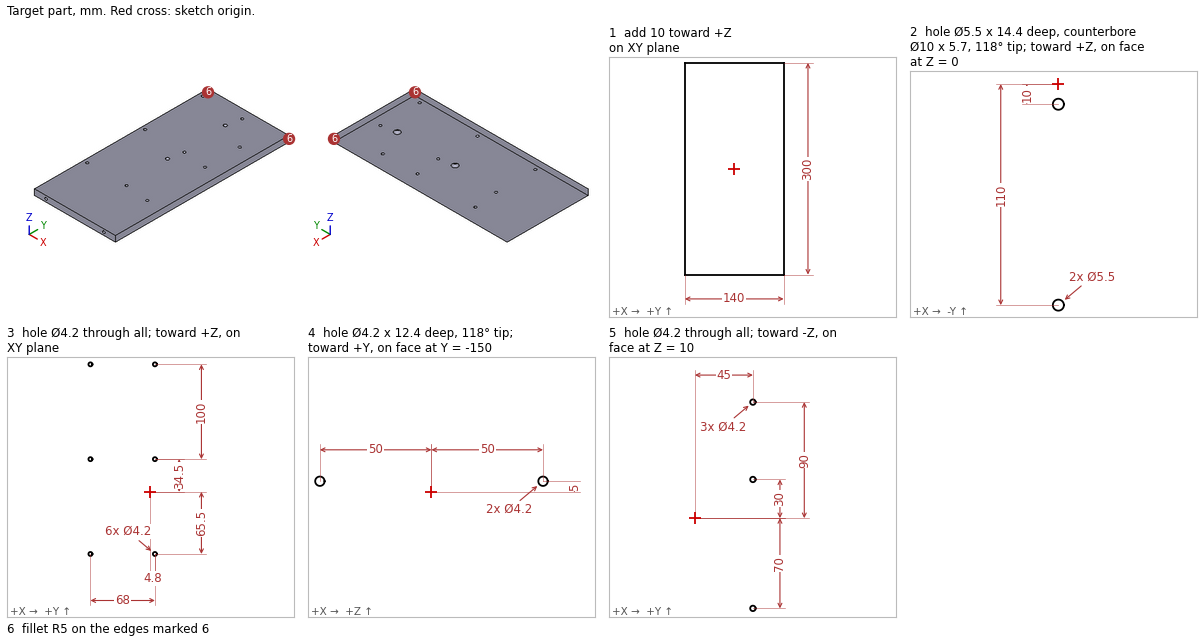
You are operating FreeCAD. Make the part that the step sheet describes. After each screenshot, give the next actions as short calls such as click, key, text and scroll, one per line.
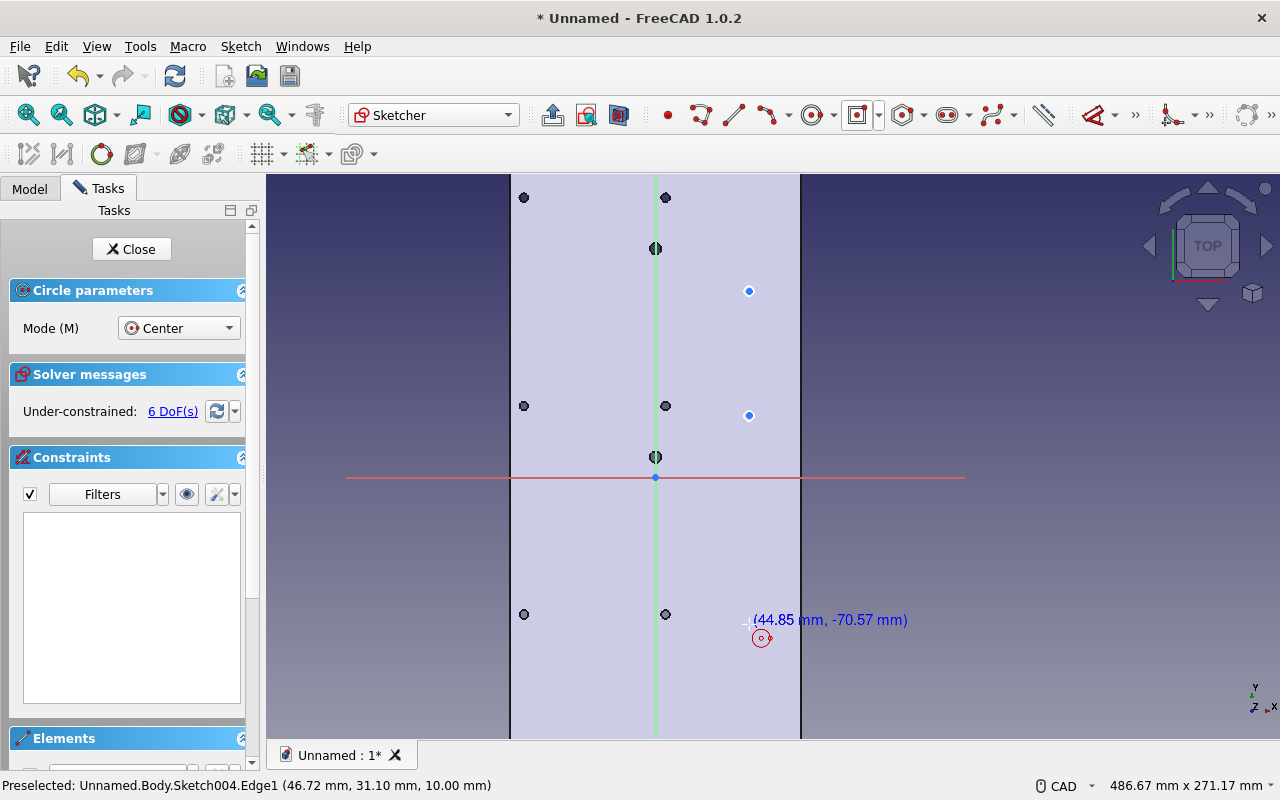
click(749, 624)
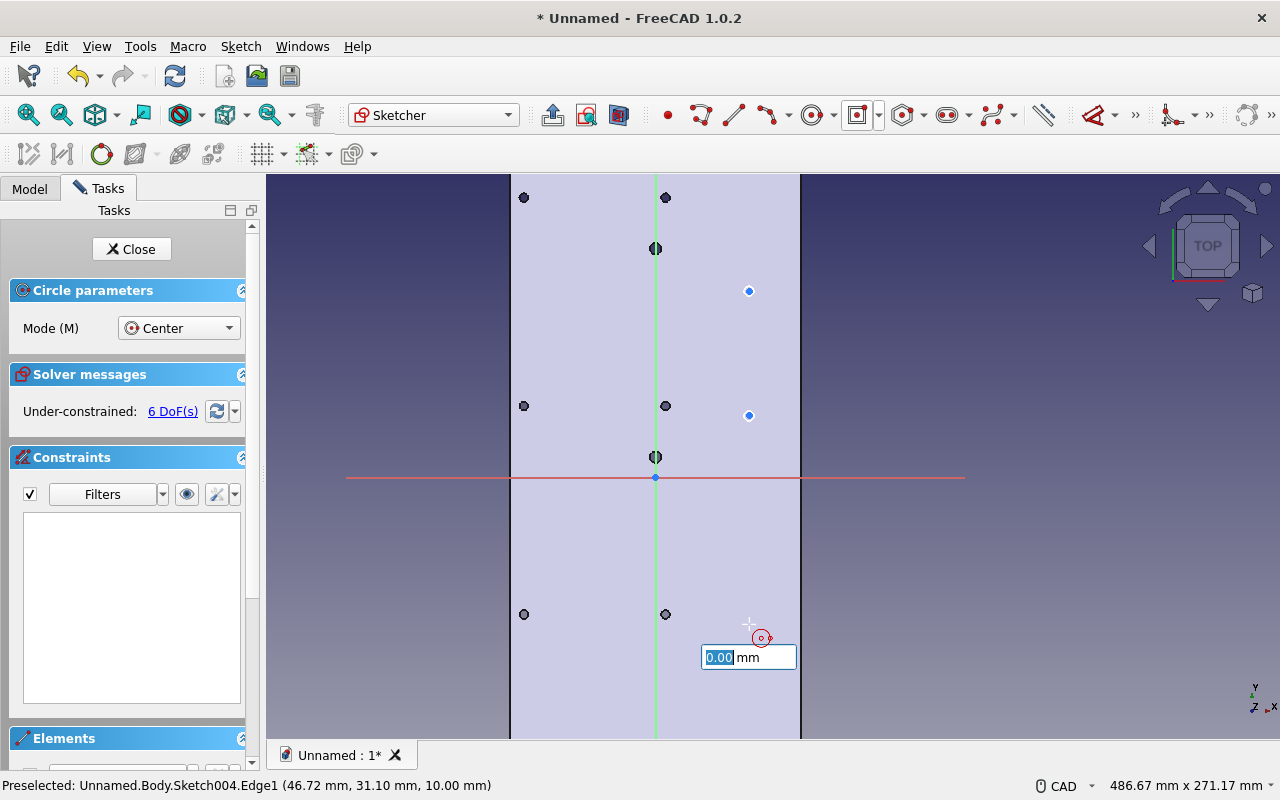
scroll(752, 621, up, 7)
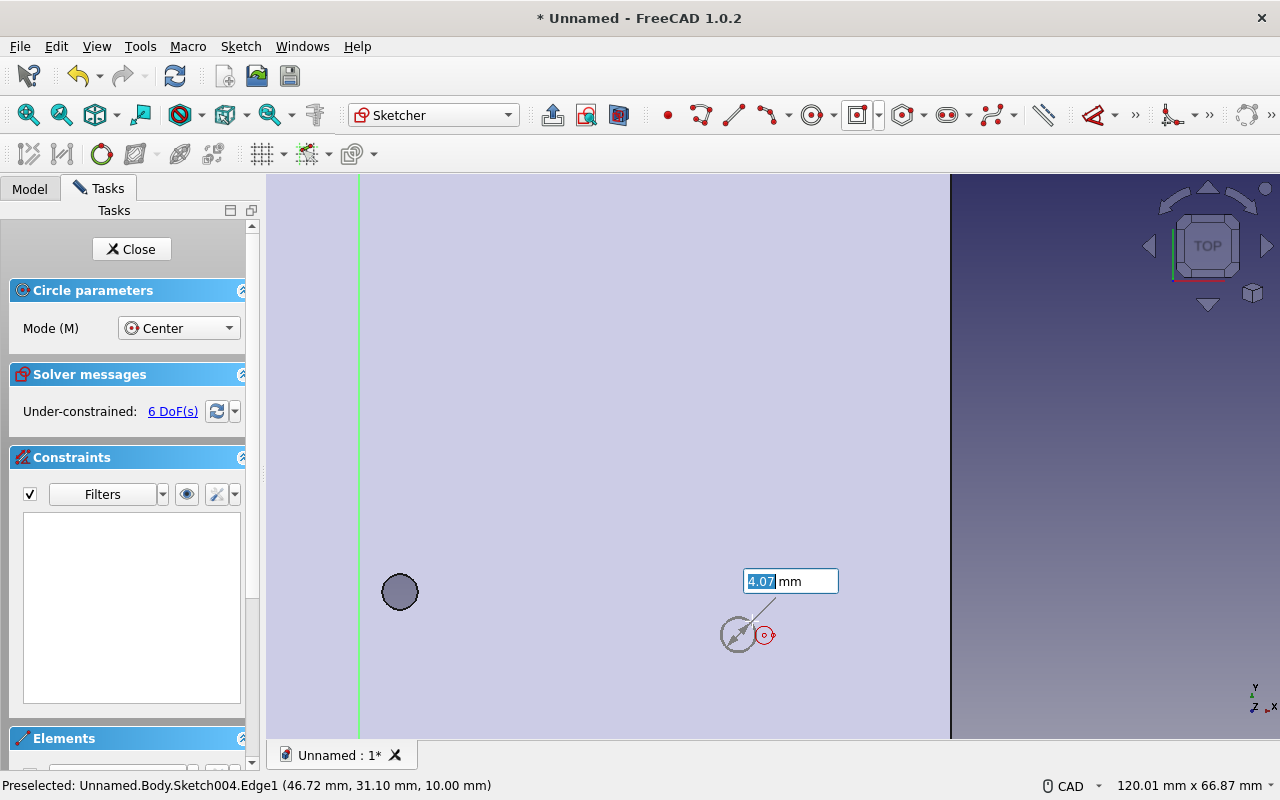
click(752, 617)
key(Escape)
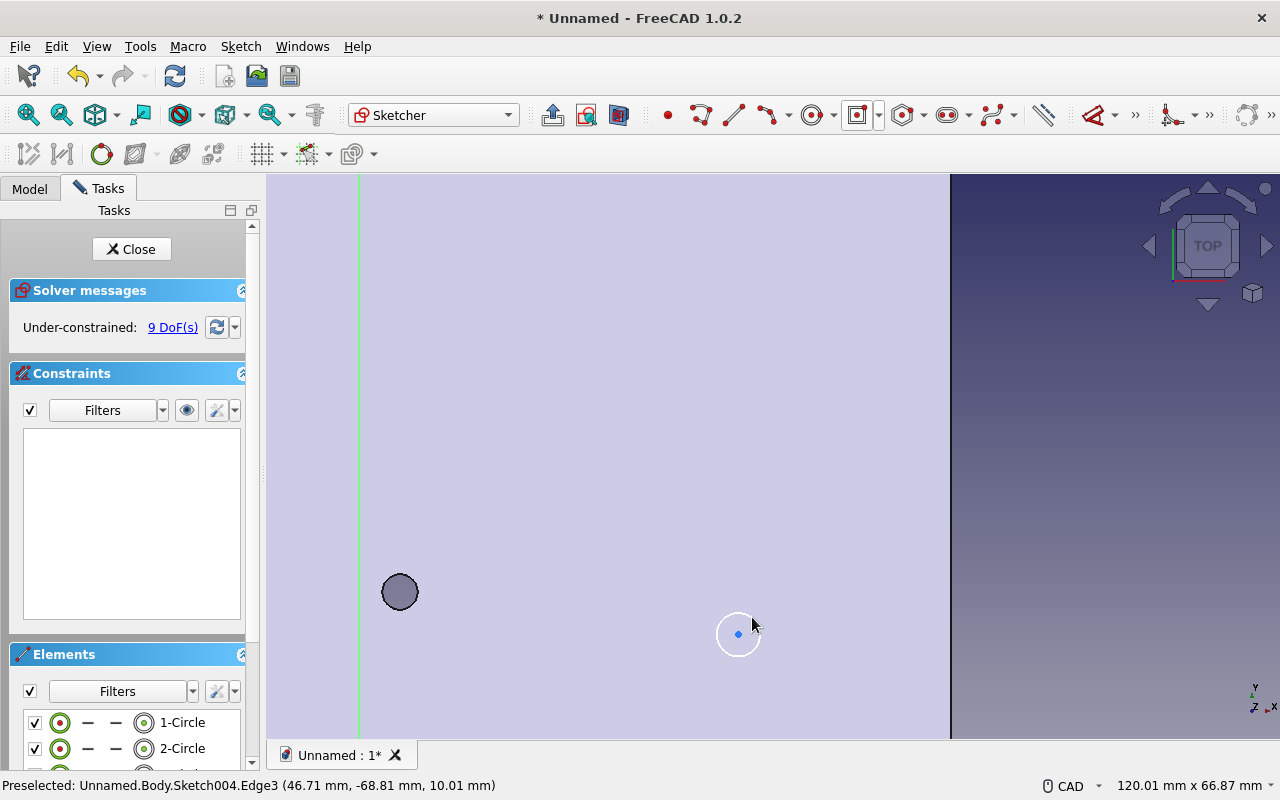
scroll(752, 621, down, 7)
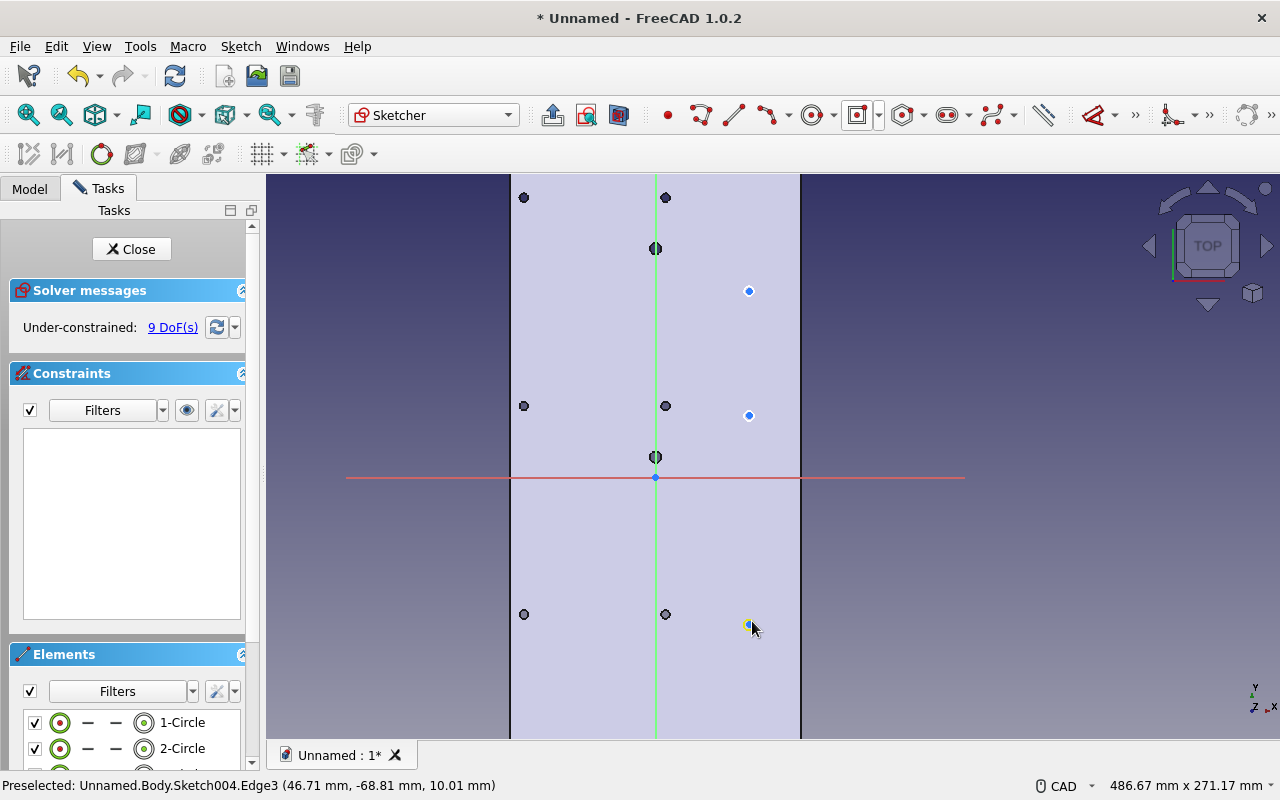
scroll(752, 288, up, 6)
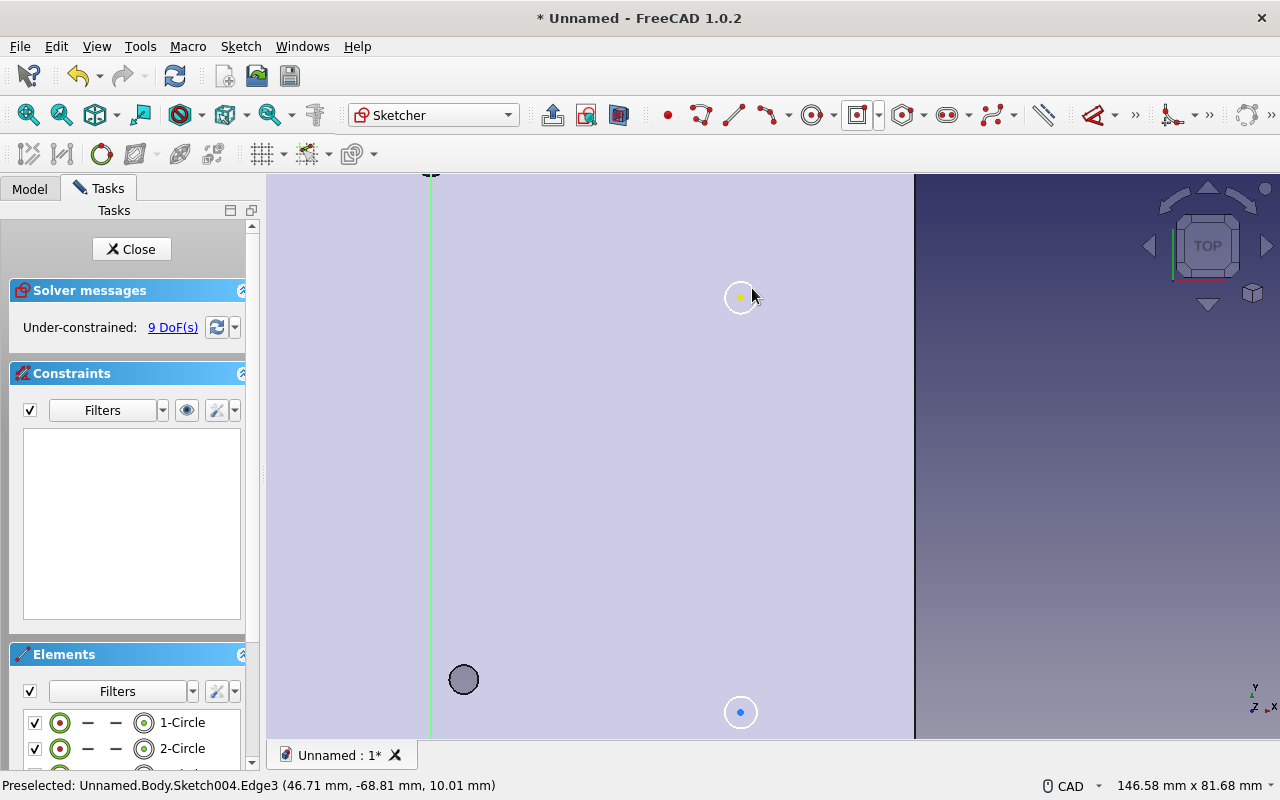
click(752, 287)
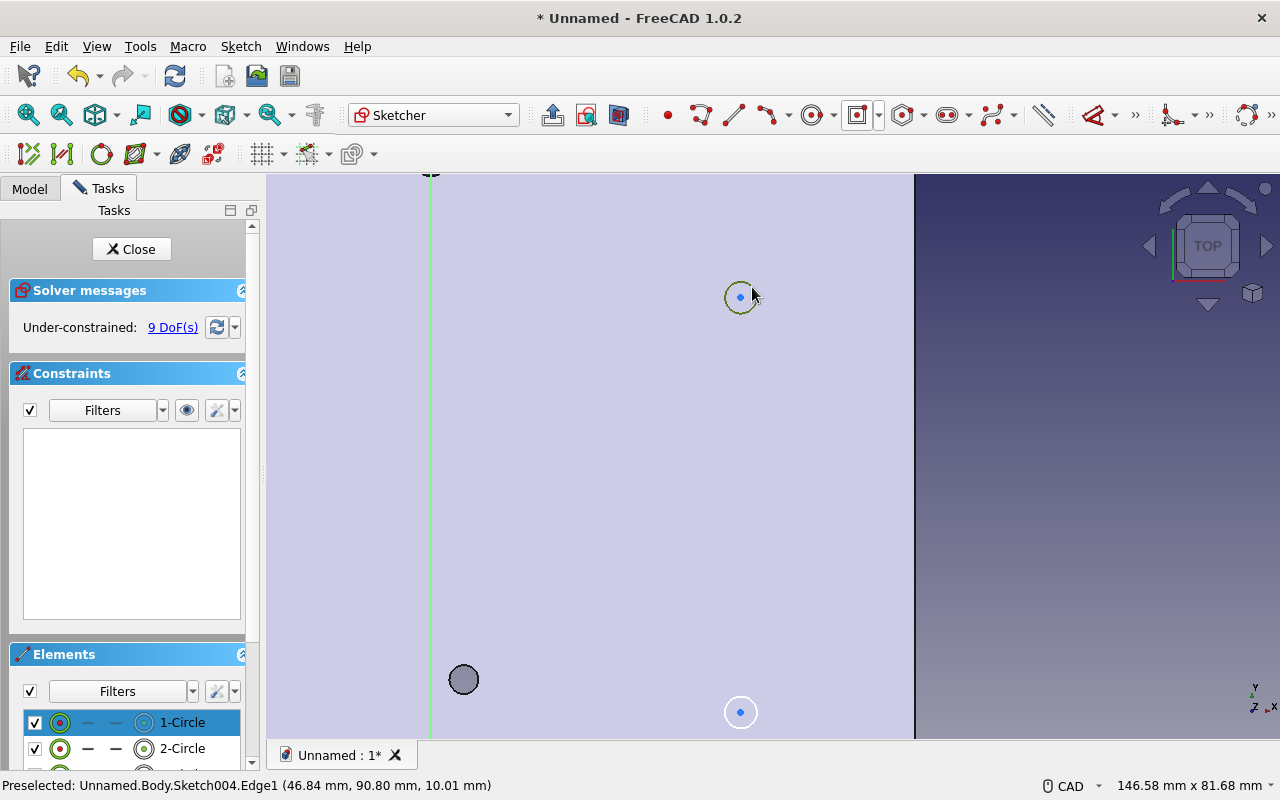
click(752, 701)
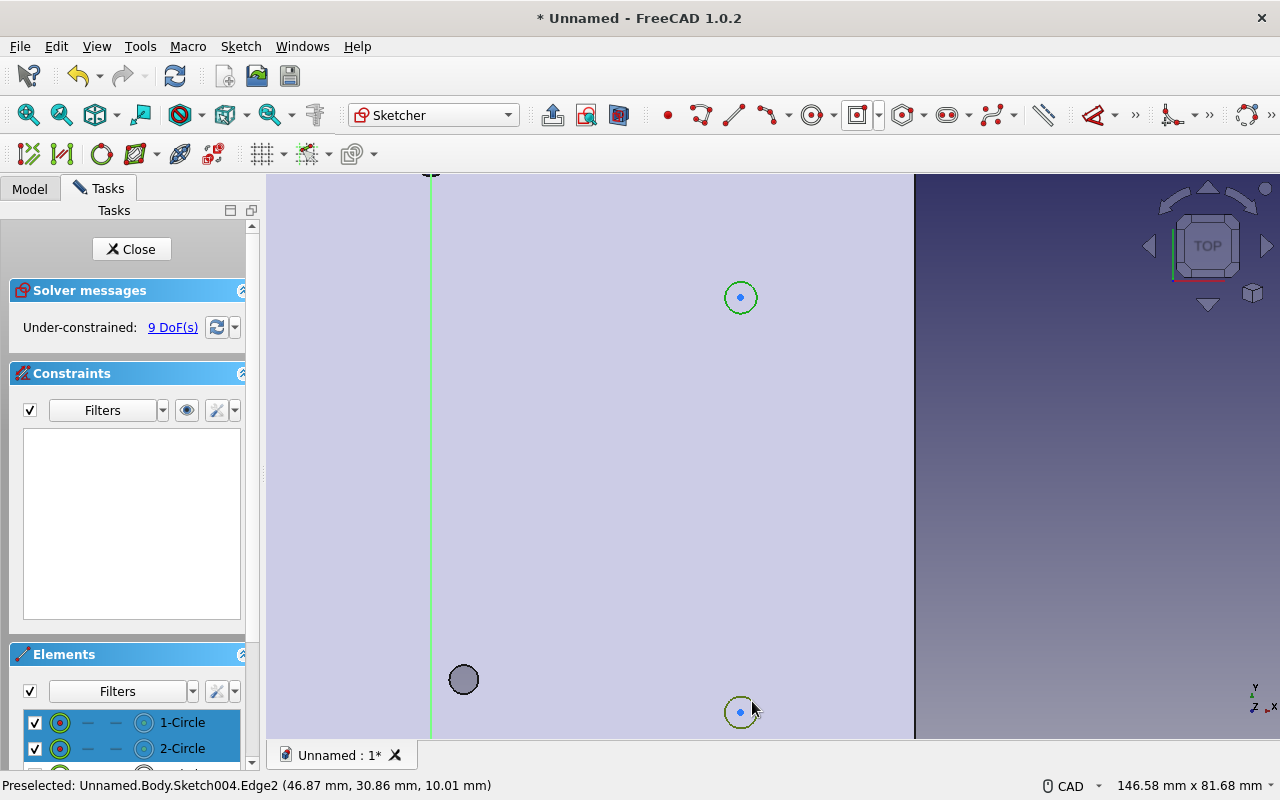
scroll(752, 287, down, 6)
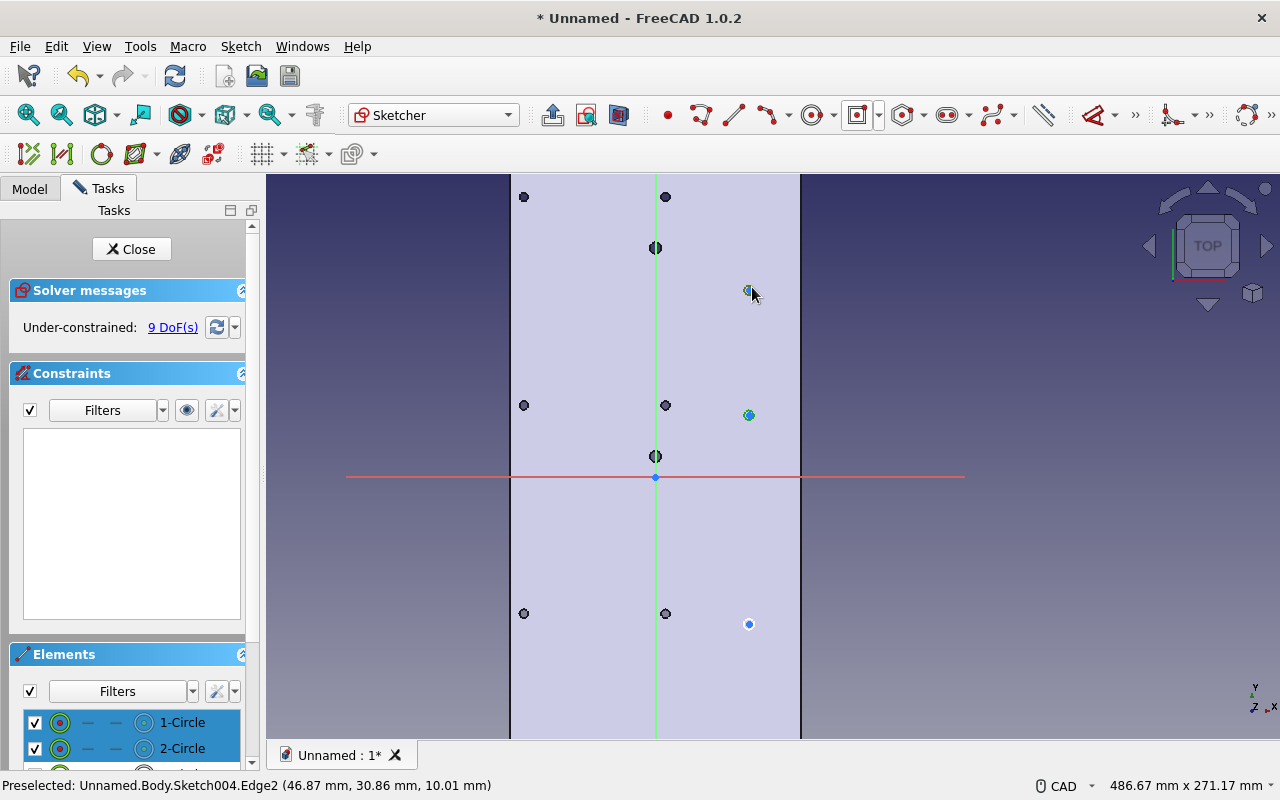
scroll(753, 621, up, 5)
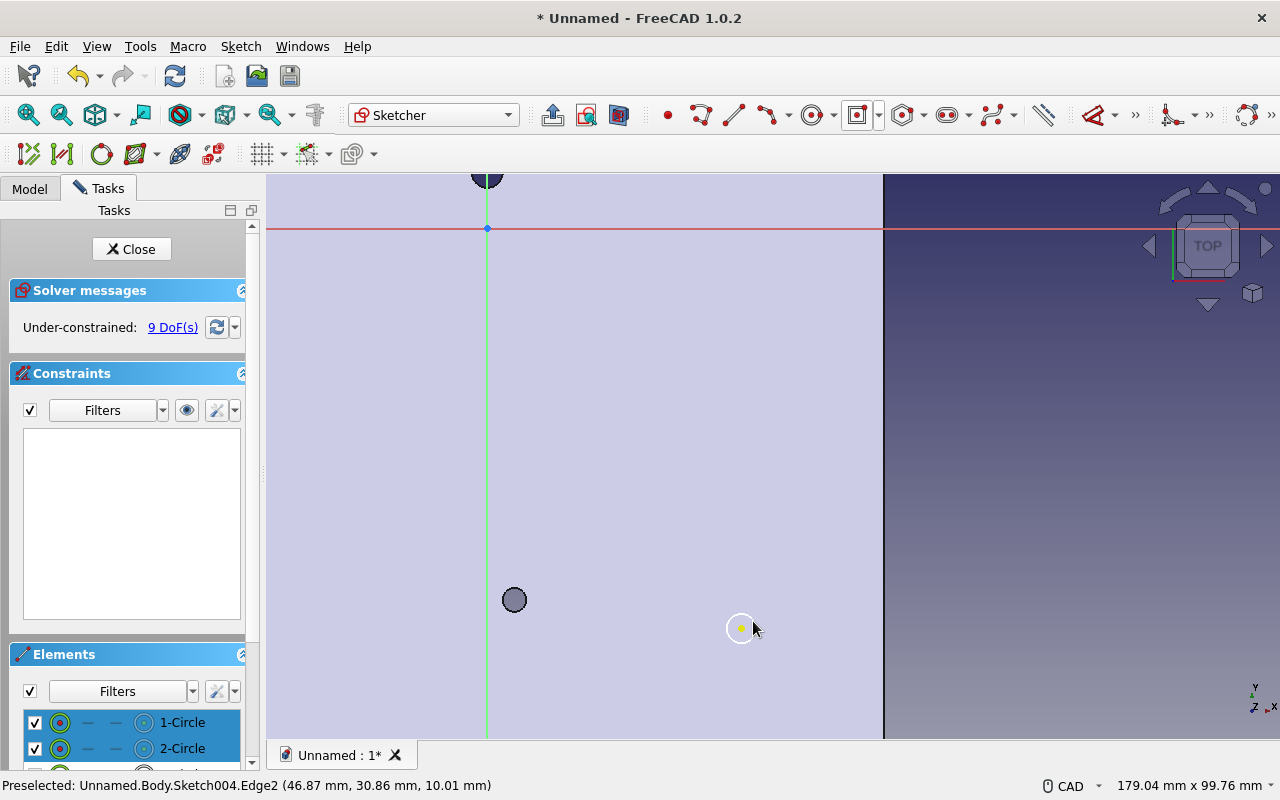
click(752, 618)